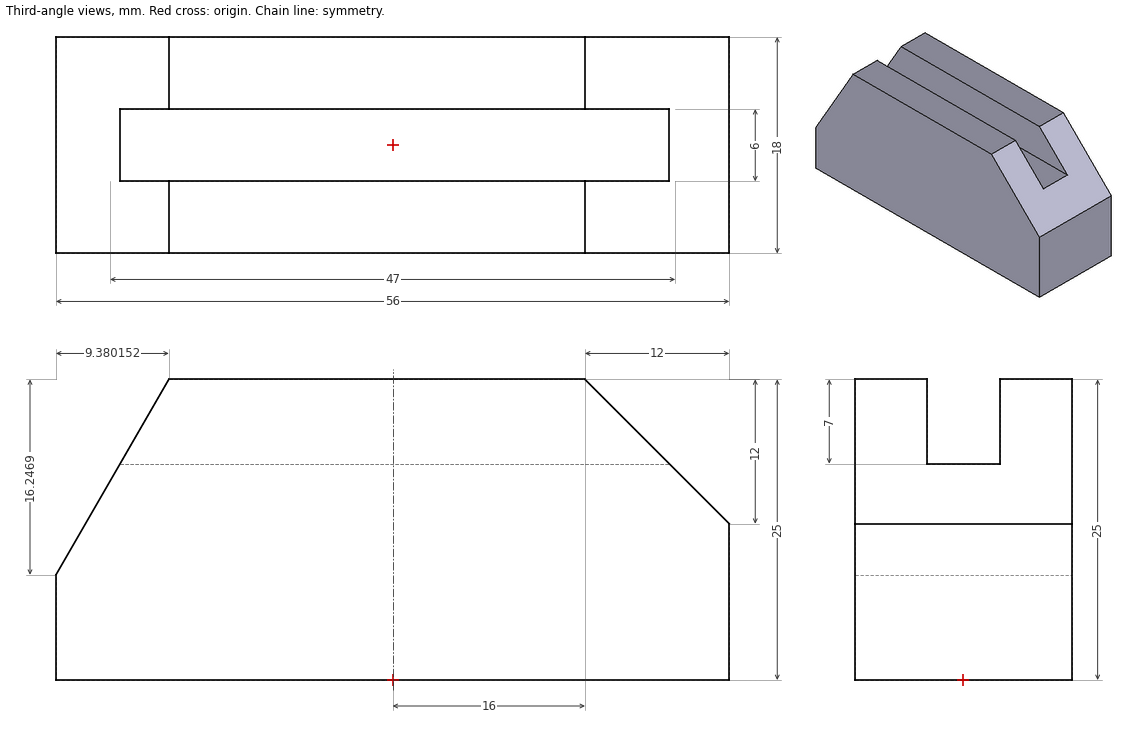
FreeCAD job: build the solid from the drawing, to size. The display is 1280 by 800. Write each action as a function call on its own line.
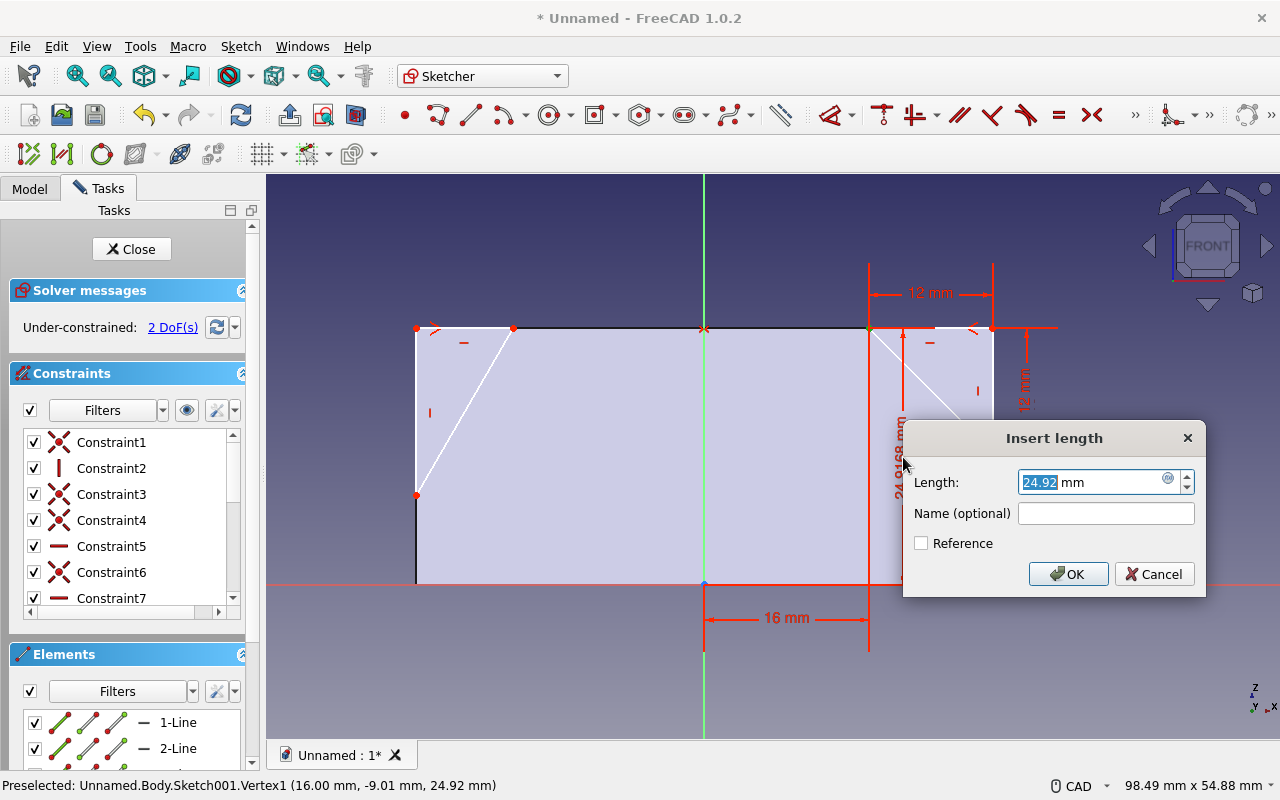
text(25)
key(Return)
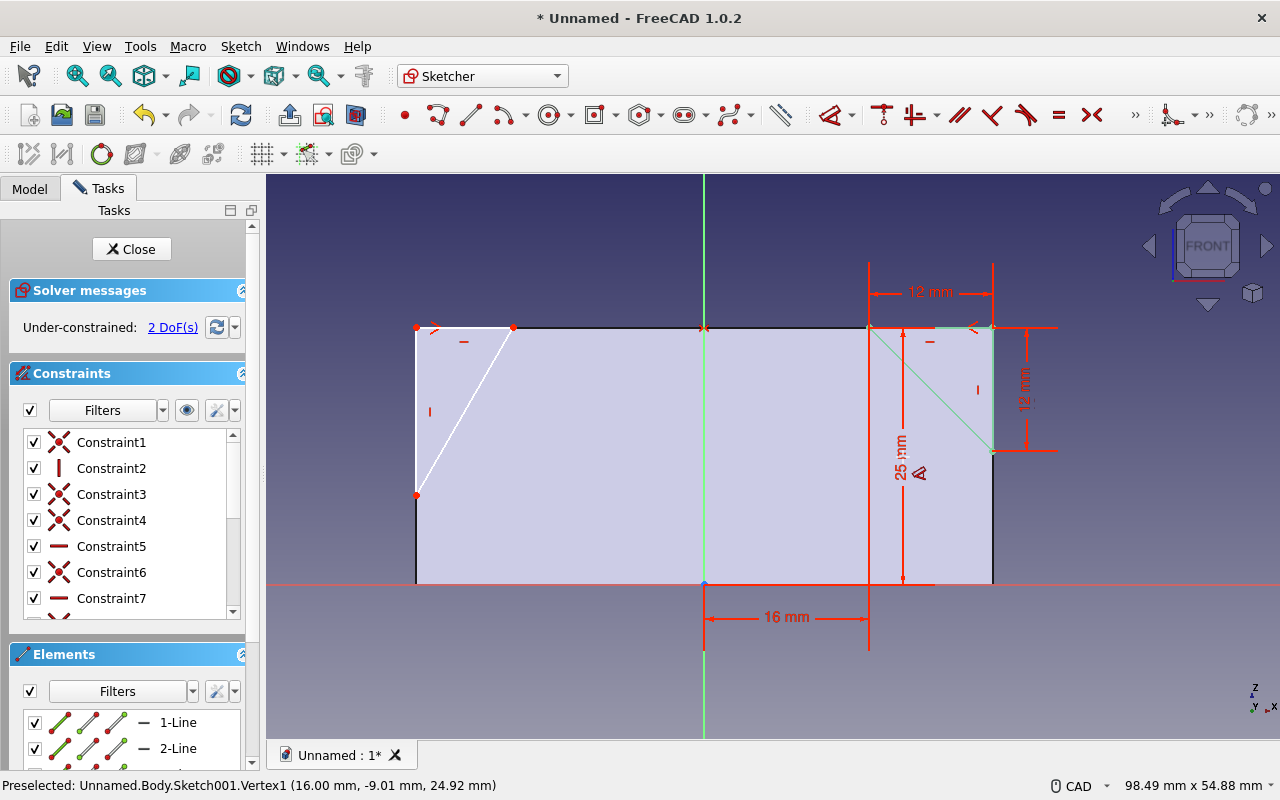
click(416, 378)
click(382, 412)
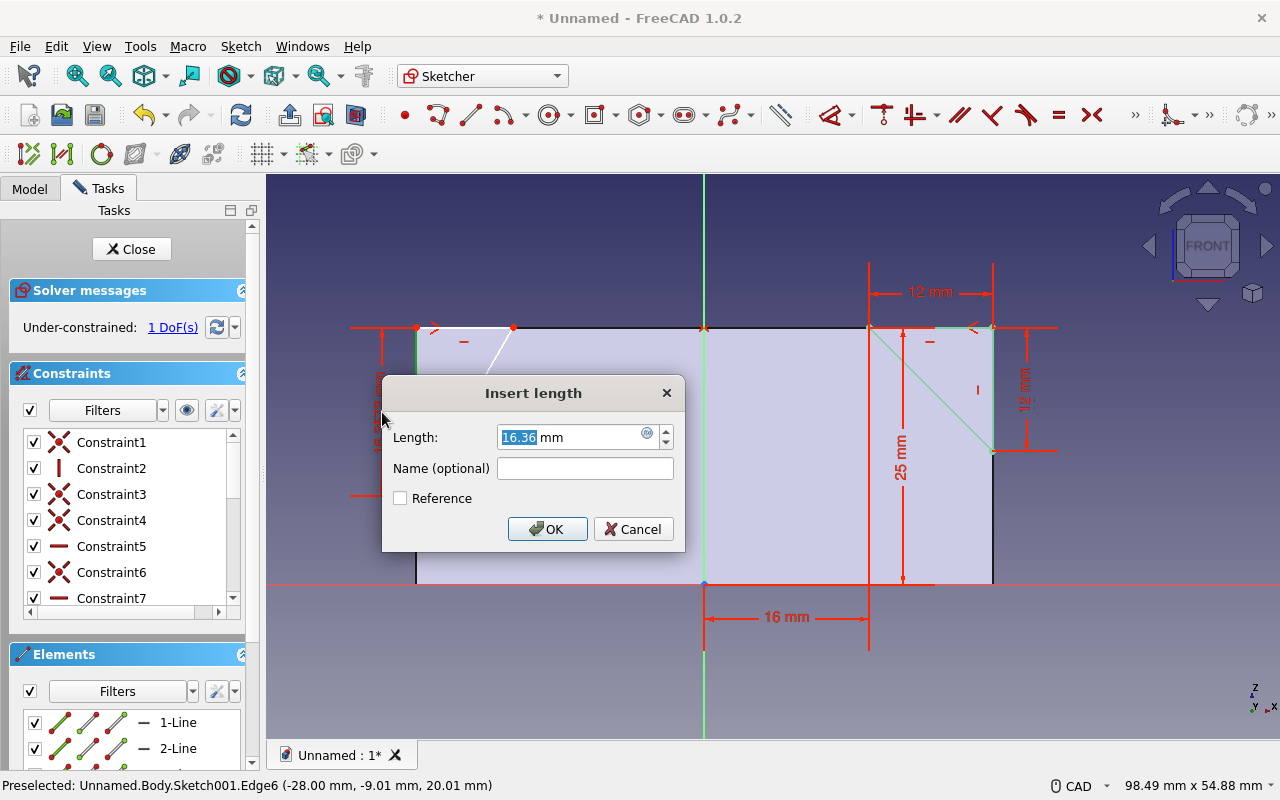
text(16.2469)
key(Return)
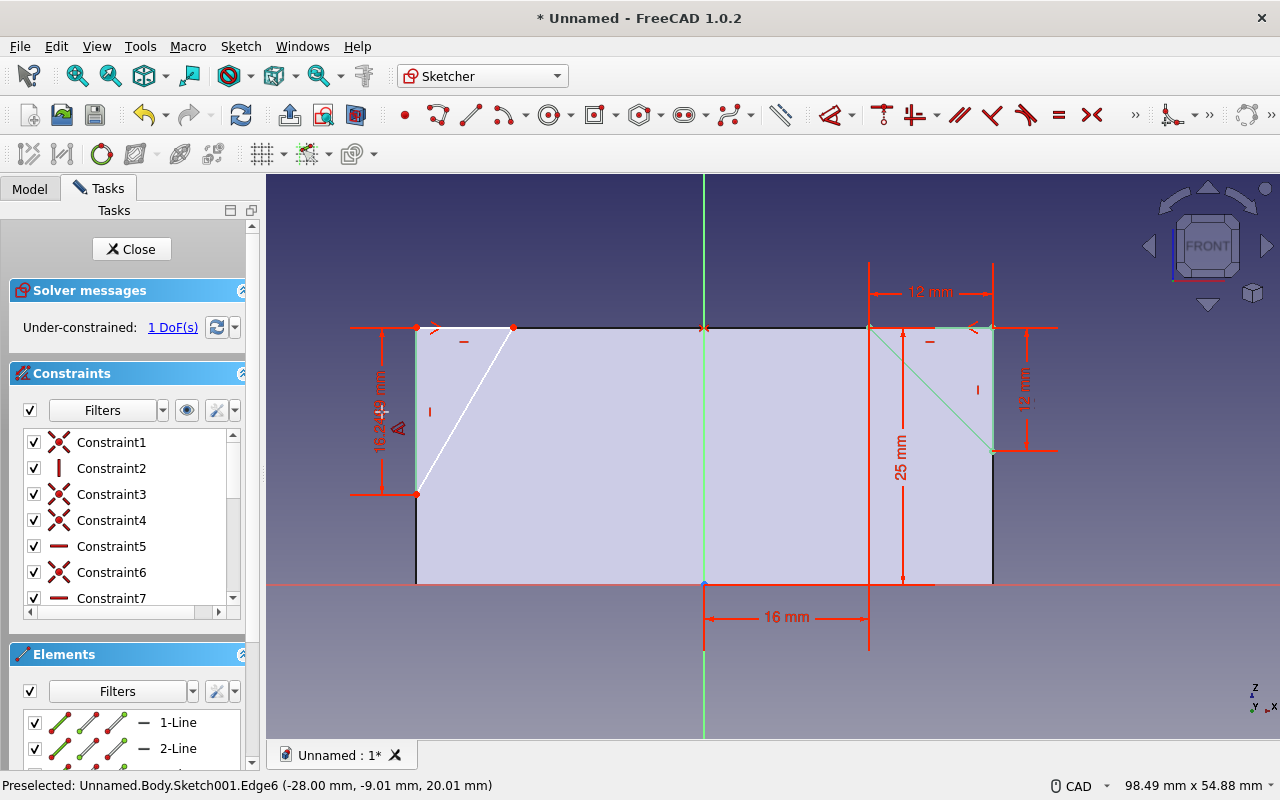
click(484, 328)
click(465, 294)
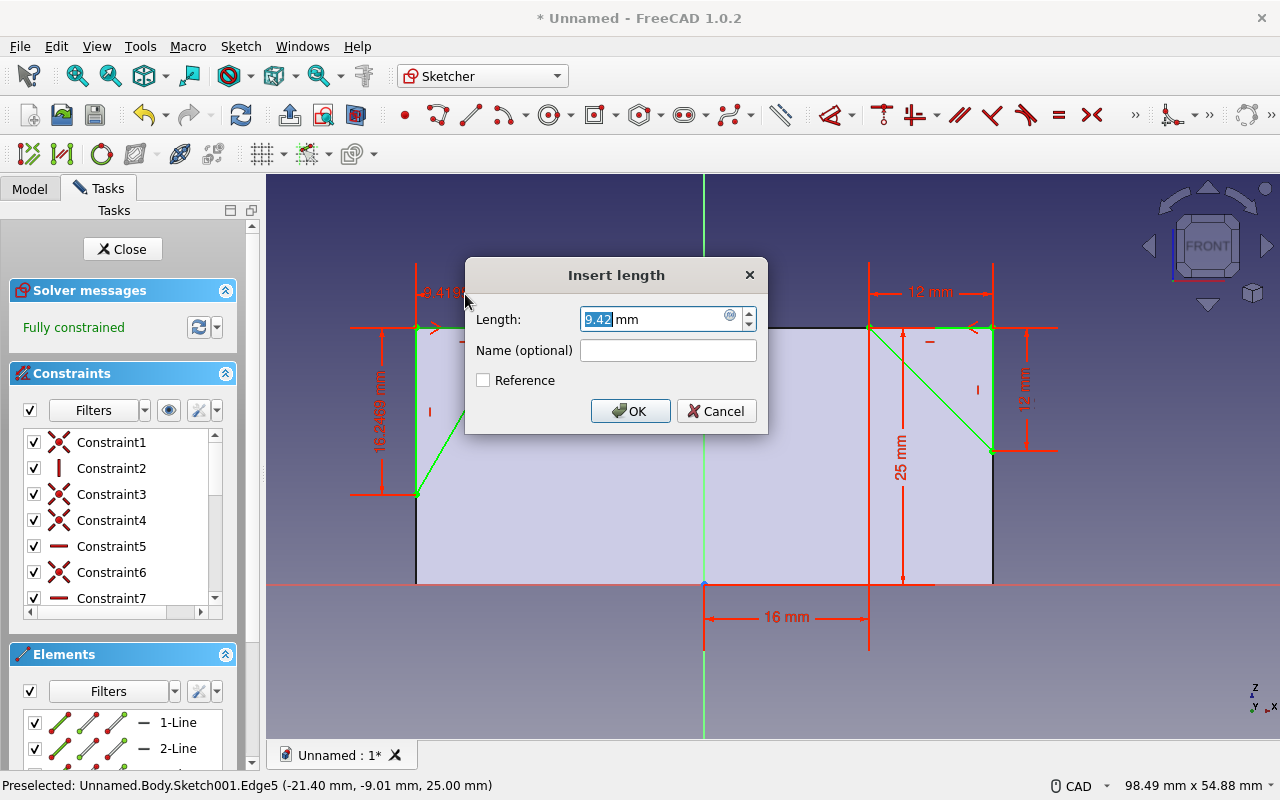
text(9.380152)
key(Return)
key(Escape)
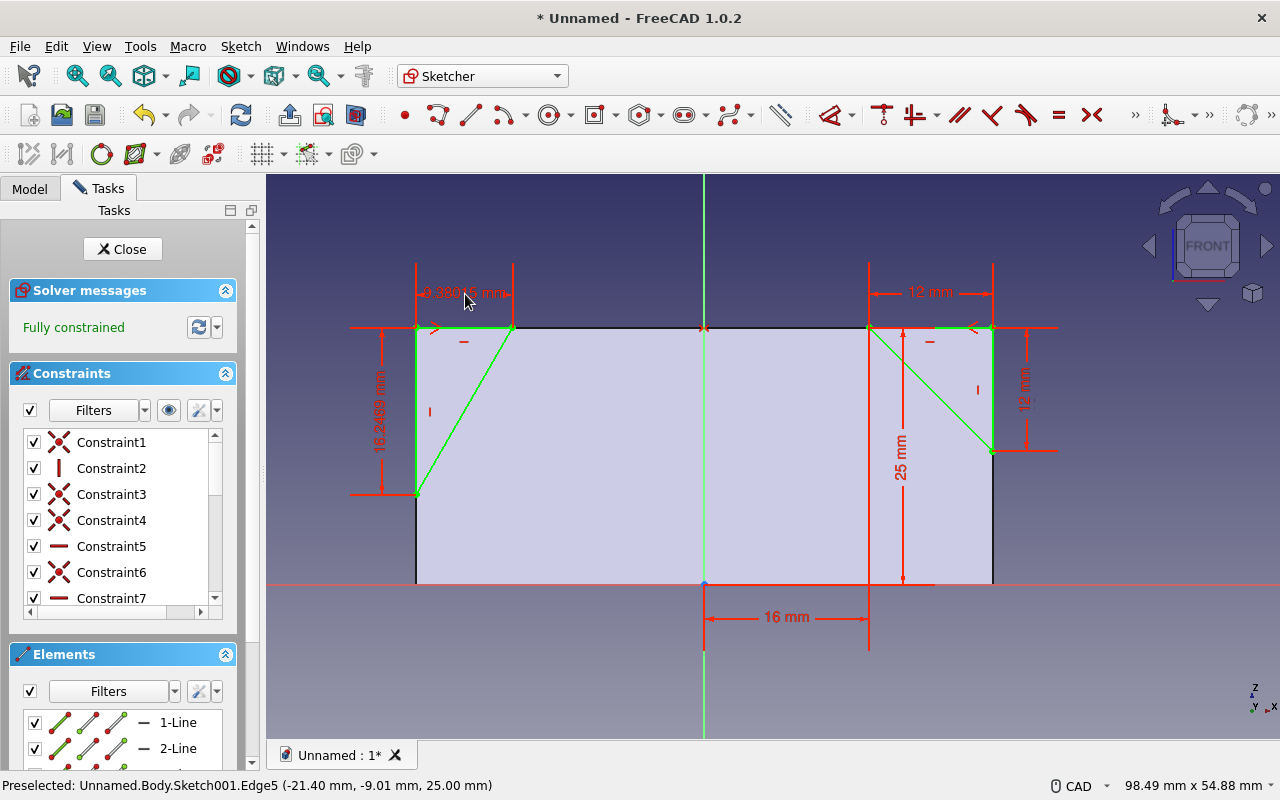
click(123, 249)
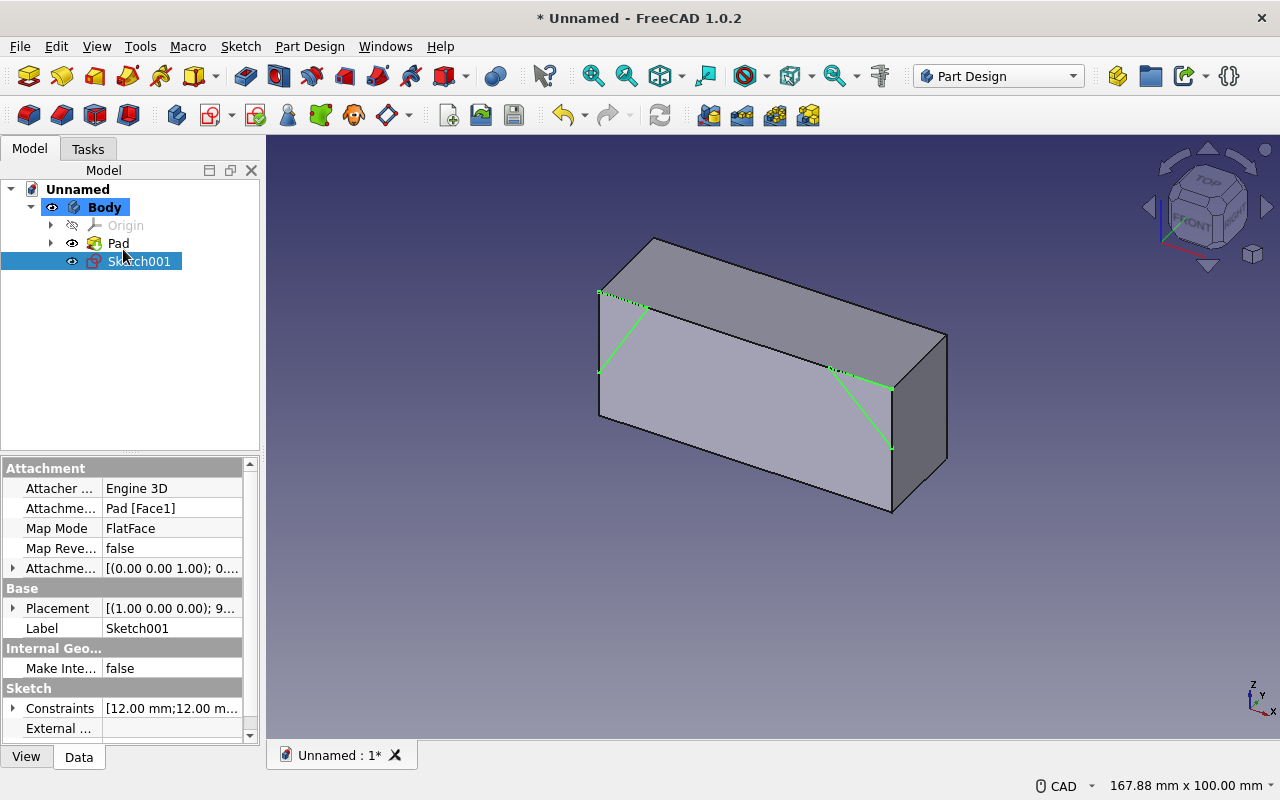
click(246, 76)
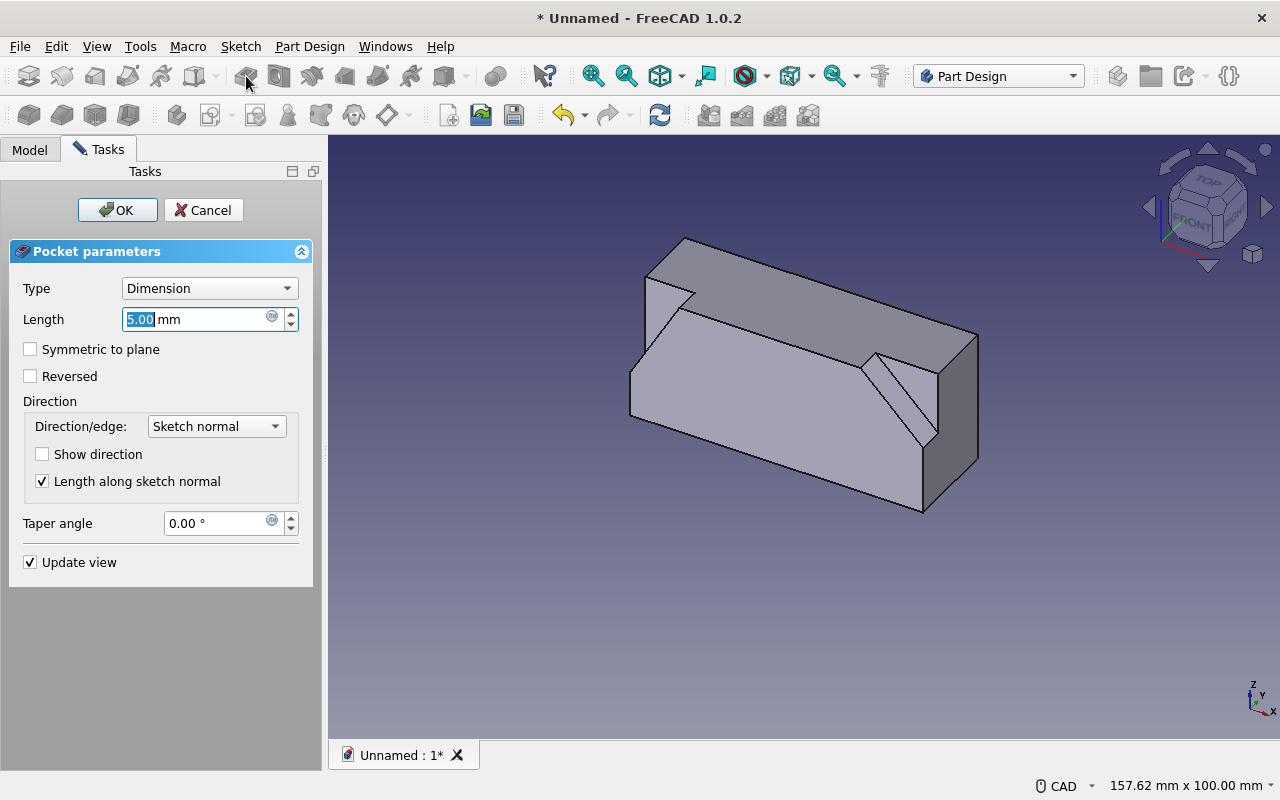
click(210, 288)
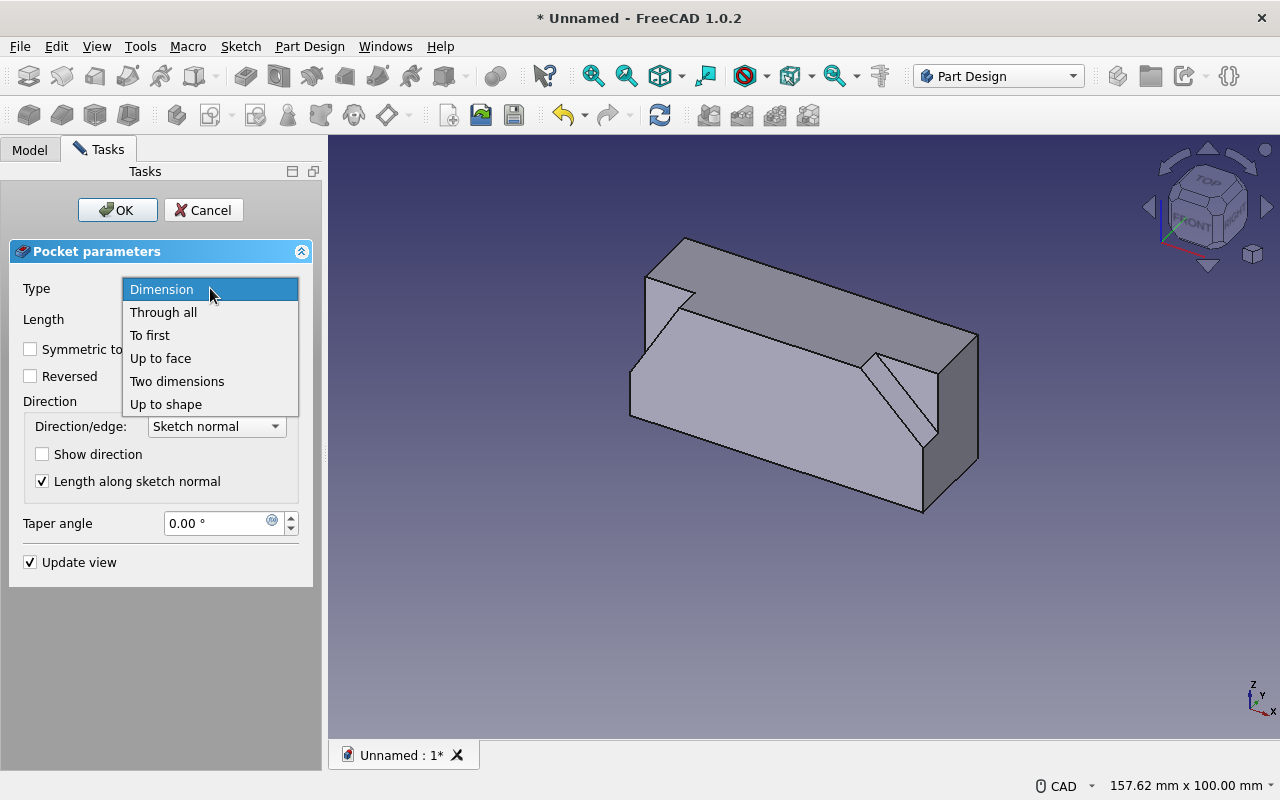
click(208, 312)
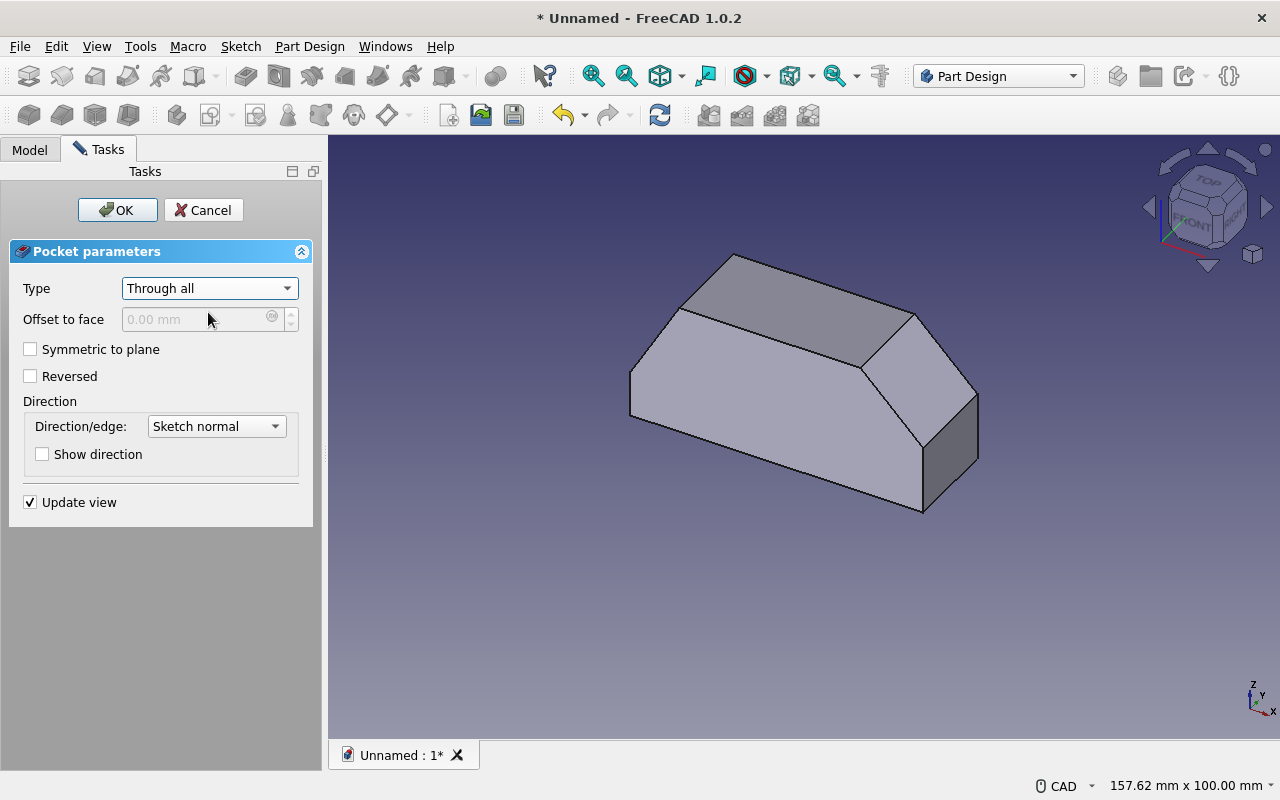
click(118, 210)